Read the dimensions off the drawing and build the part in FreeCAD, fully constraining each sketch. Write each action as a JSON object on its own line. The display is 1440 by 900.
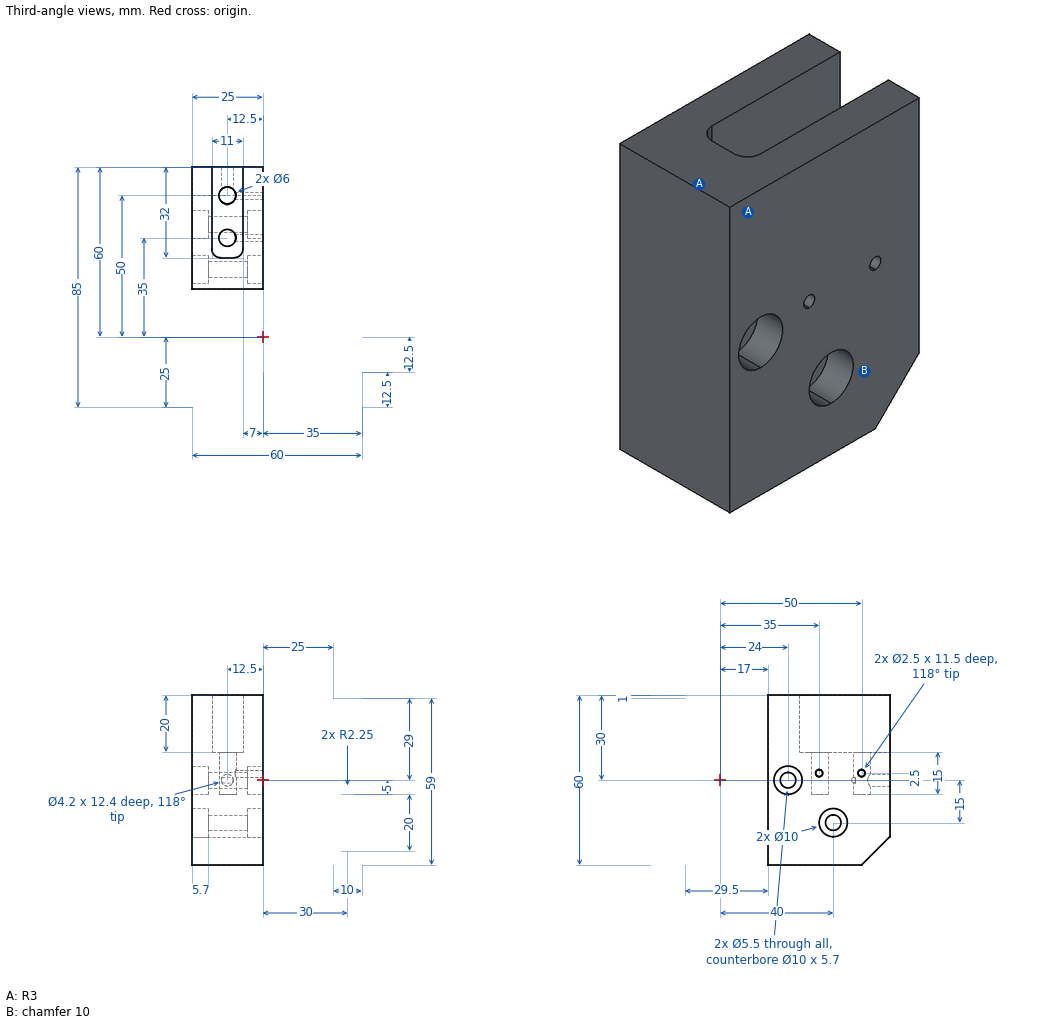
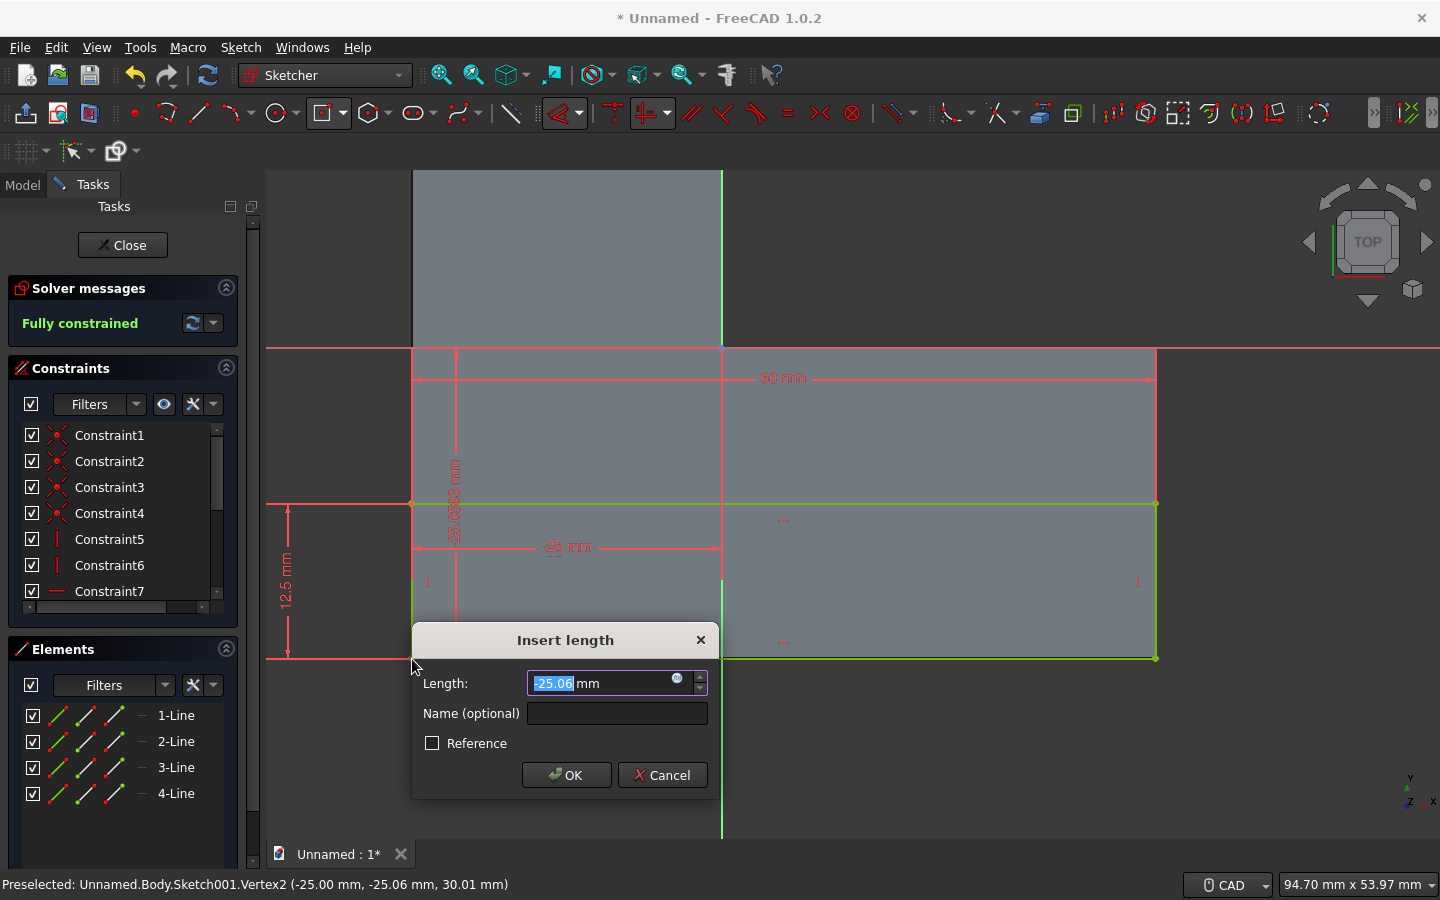
{"action": "type", "text": "-25"}
{"action": "key", "text": "Return"}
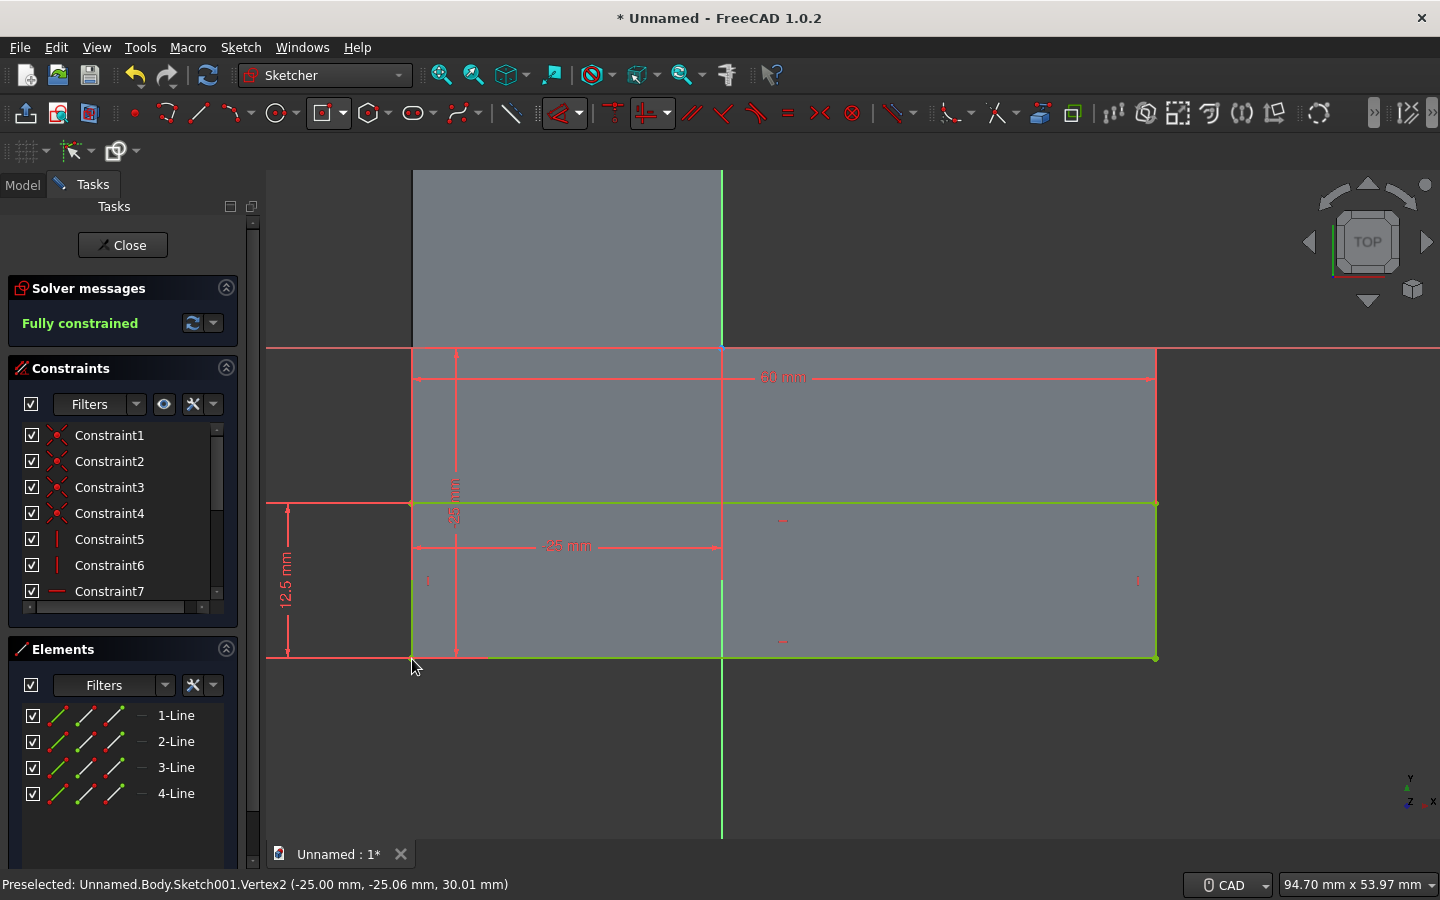
{"action": "left_click", "coordinate": [123, 245]}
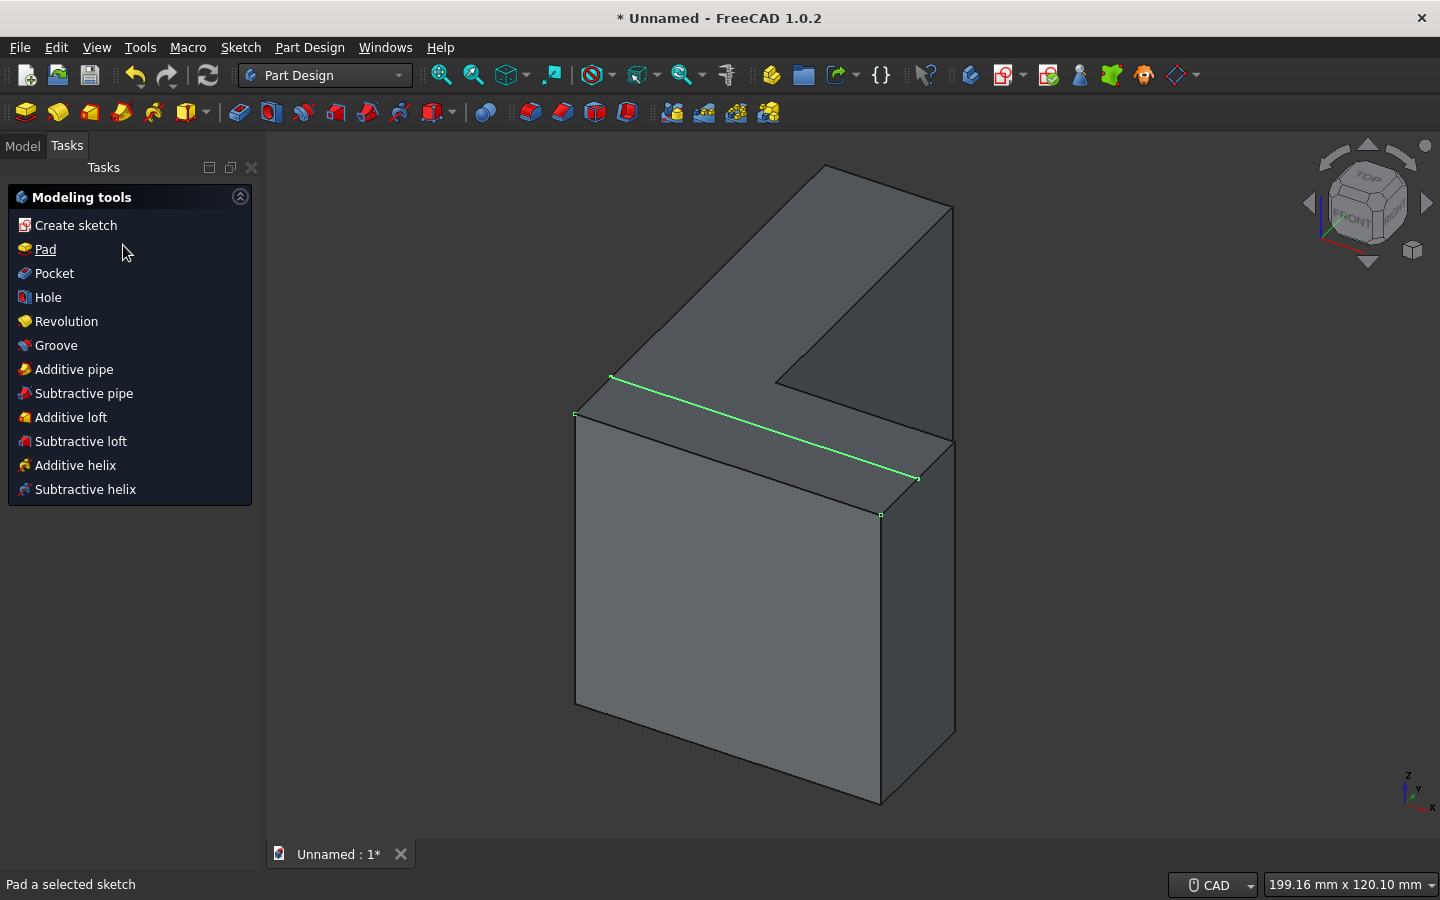
{"action": "left_click", "coordinate": [240, 112]}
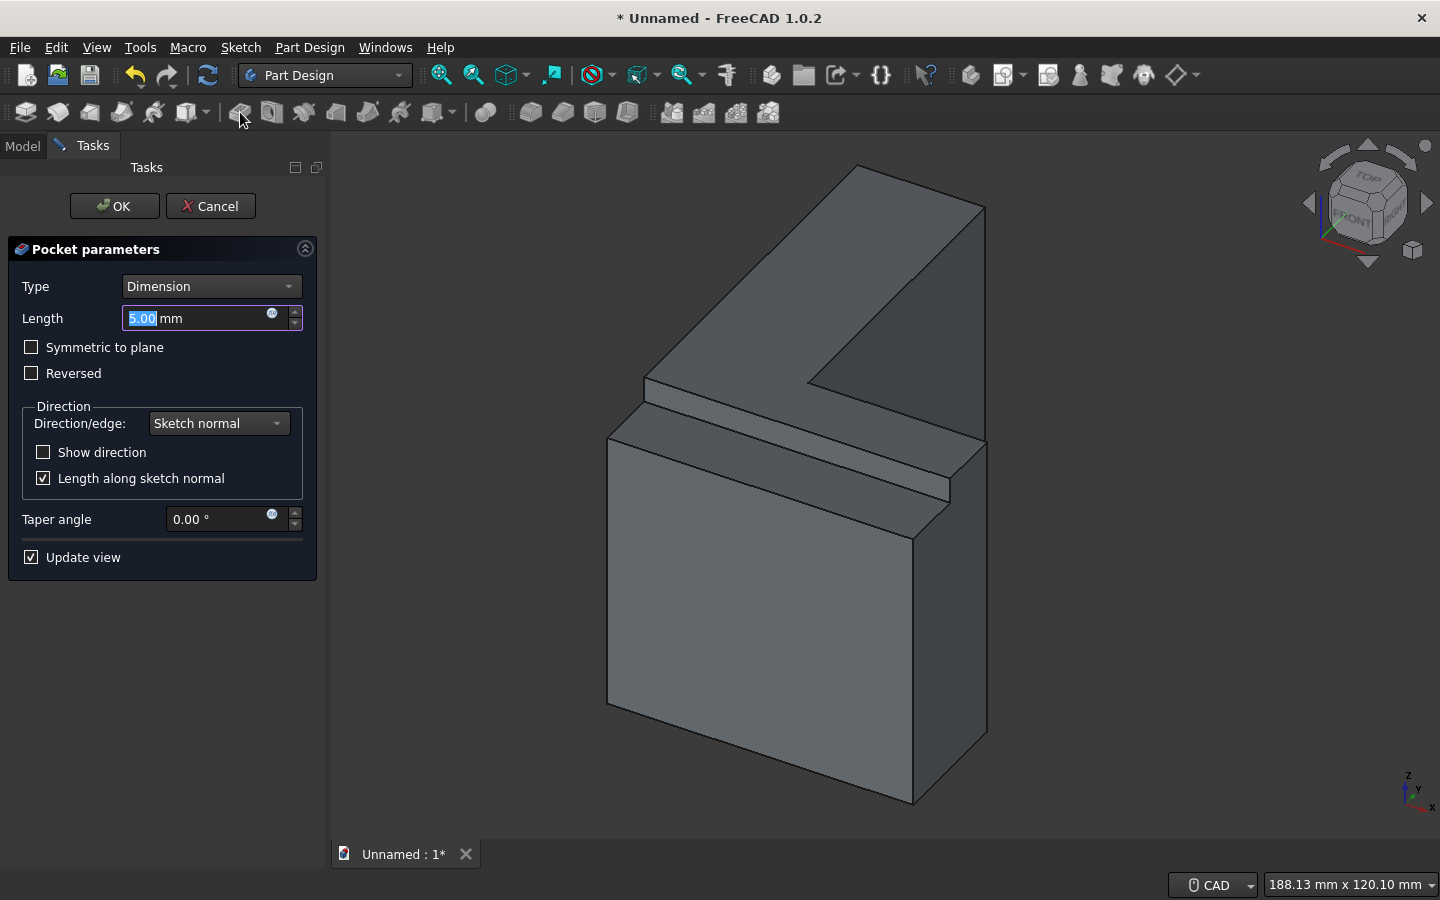
{"action": "left_click", "coordinate": [212, 286]}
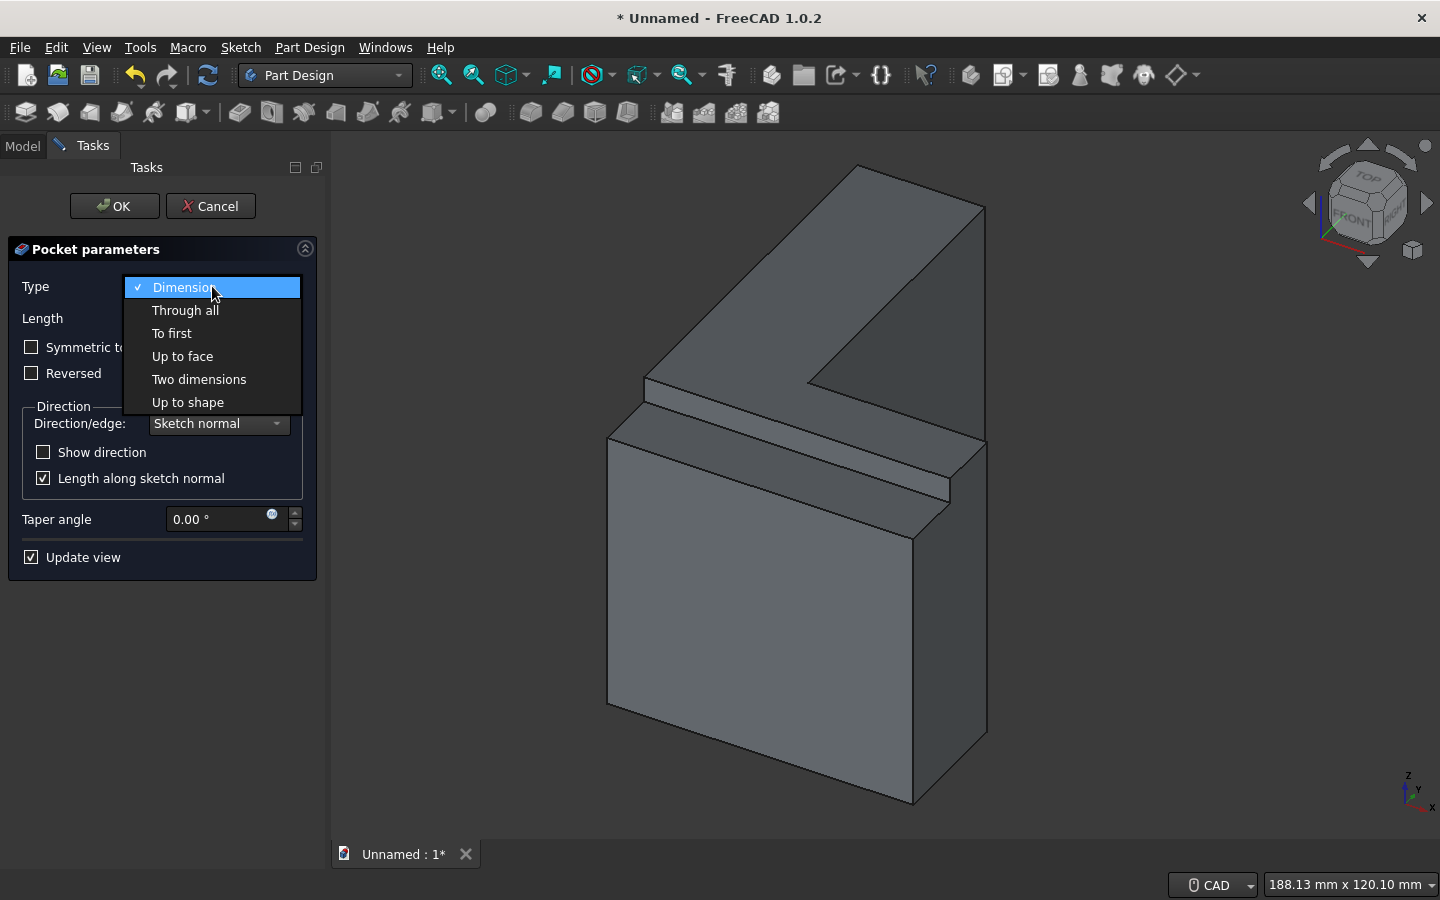
{"action": "left_click", "coordinate": [212, 310]}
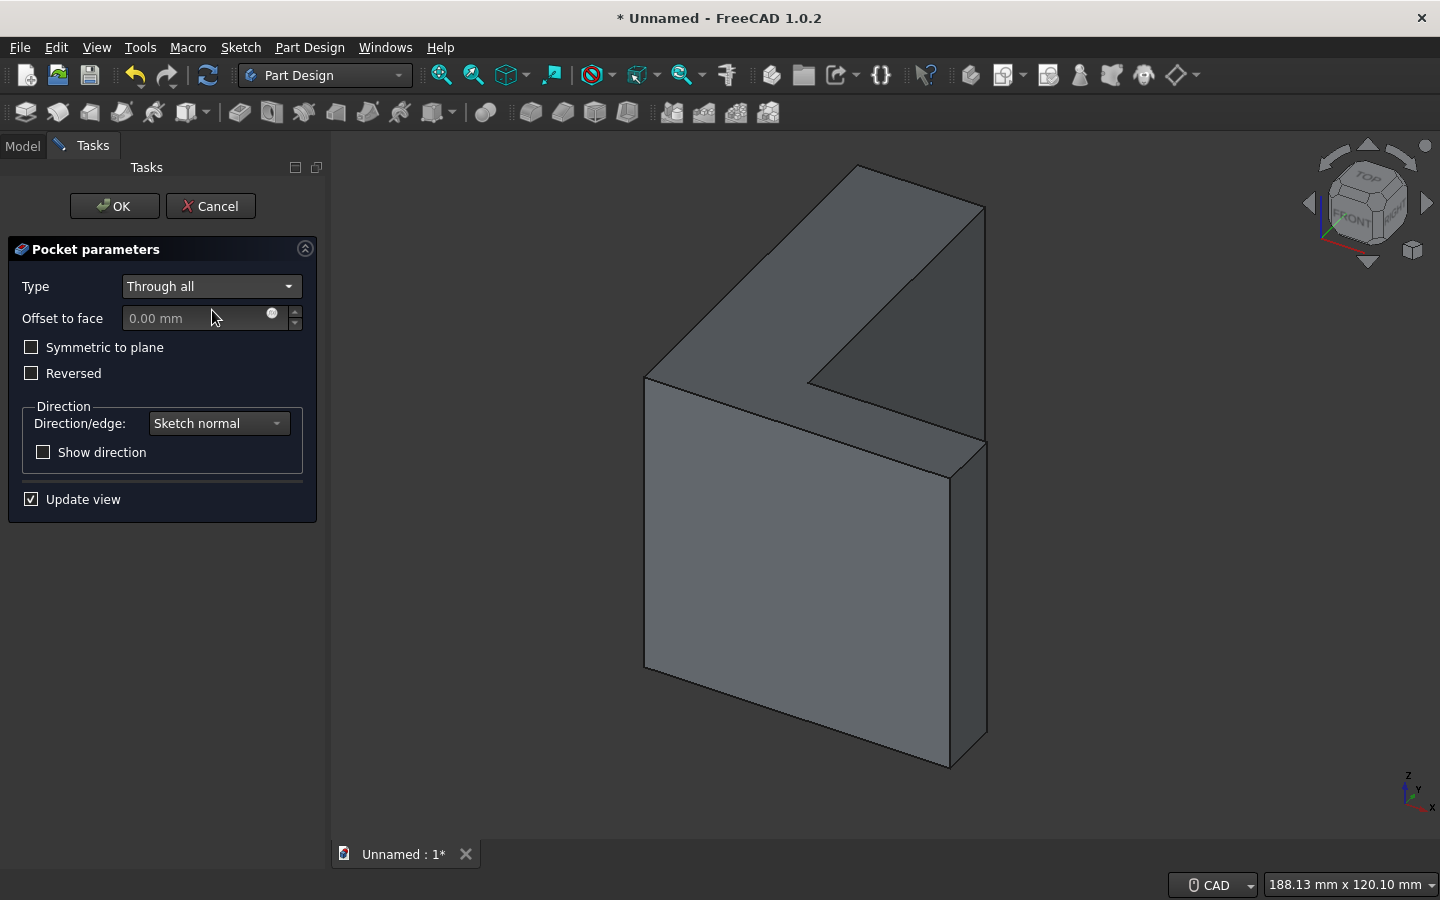
{"action": "left_click", "coordinate": [115, 206]}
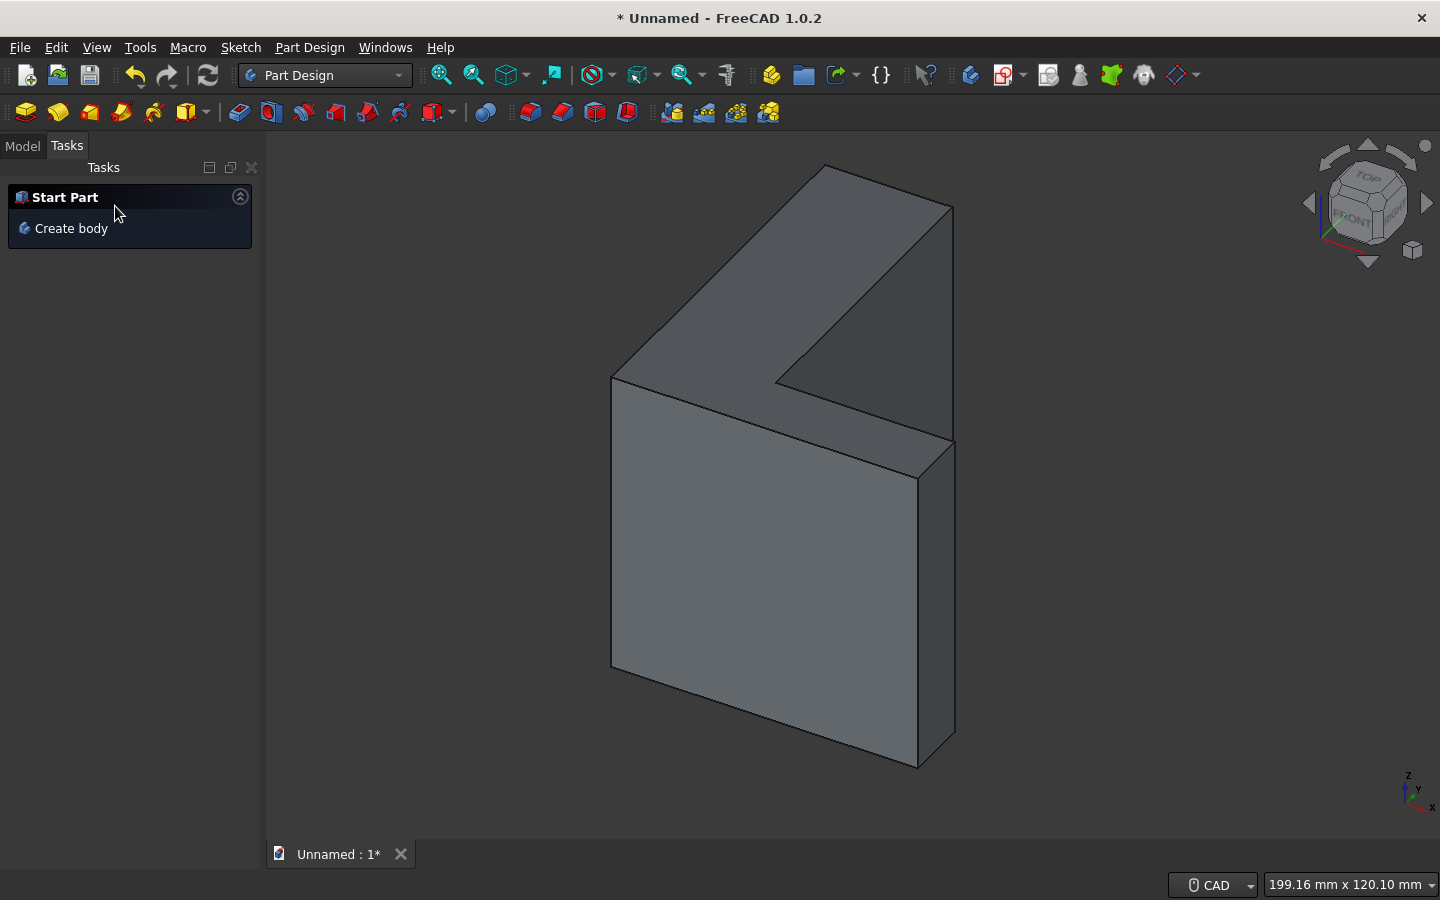
{"action": "left_click", "coordinate": [845, 231]}